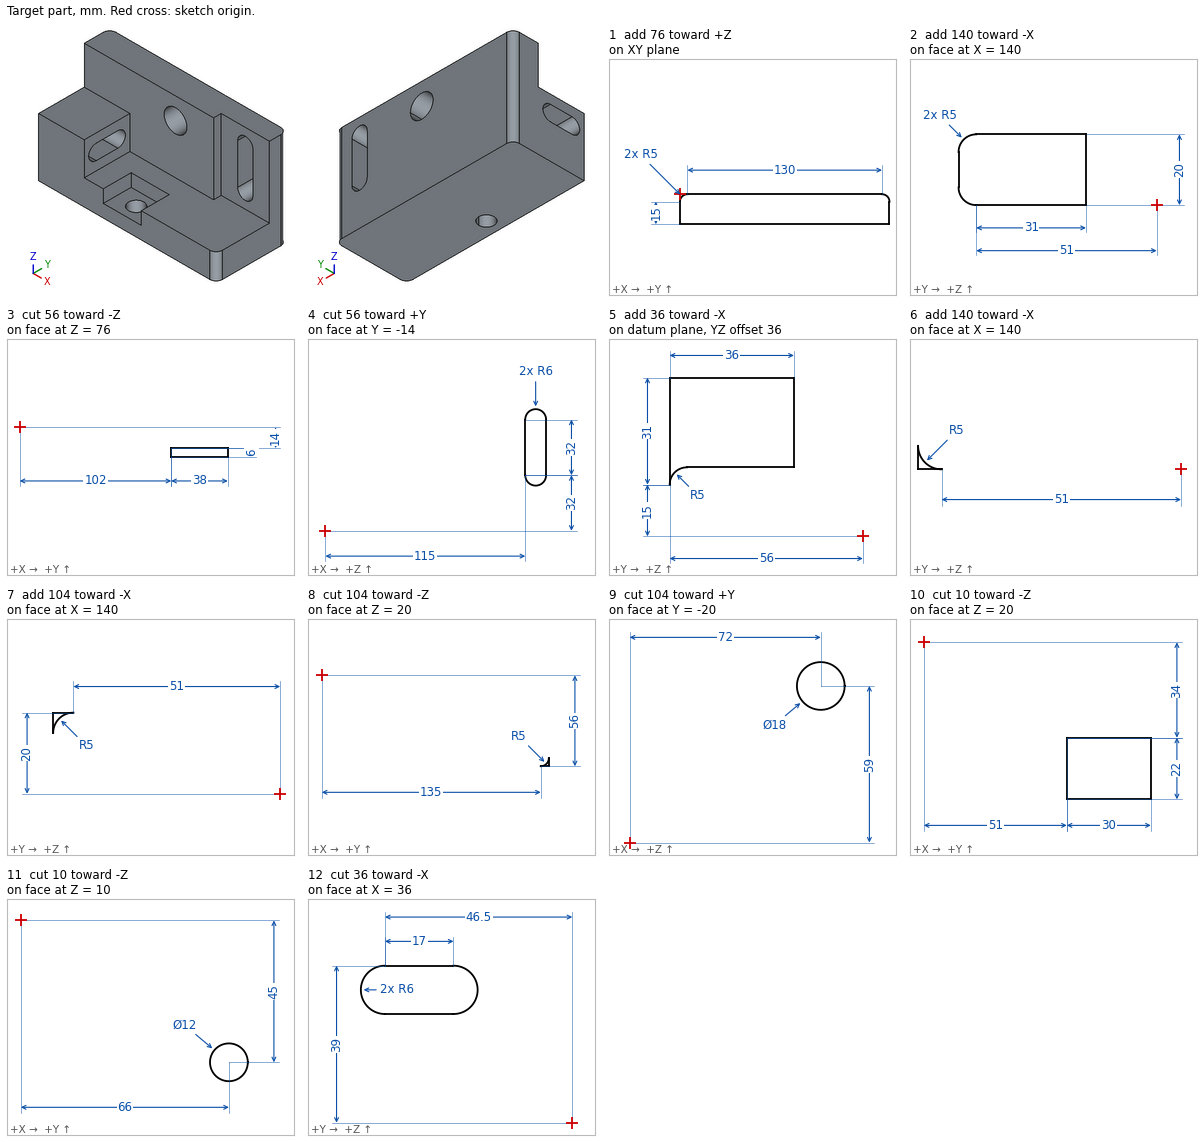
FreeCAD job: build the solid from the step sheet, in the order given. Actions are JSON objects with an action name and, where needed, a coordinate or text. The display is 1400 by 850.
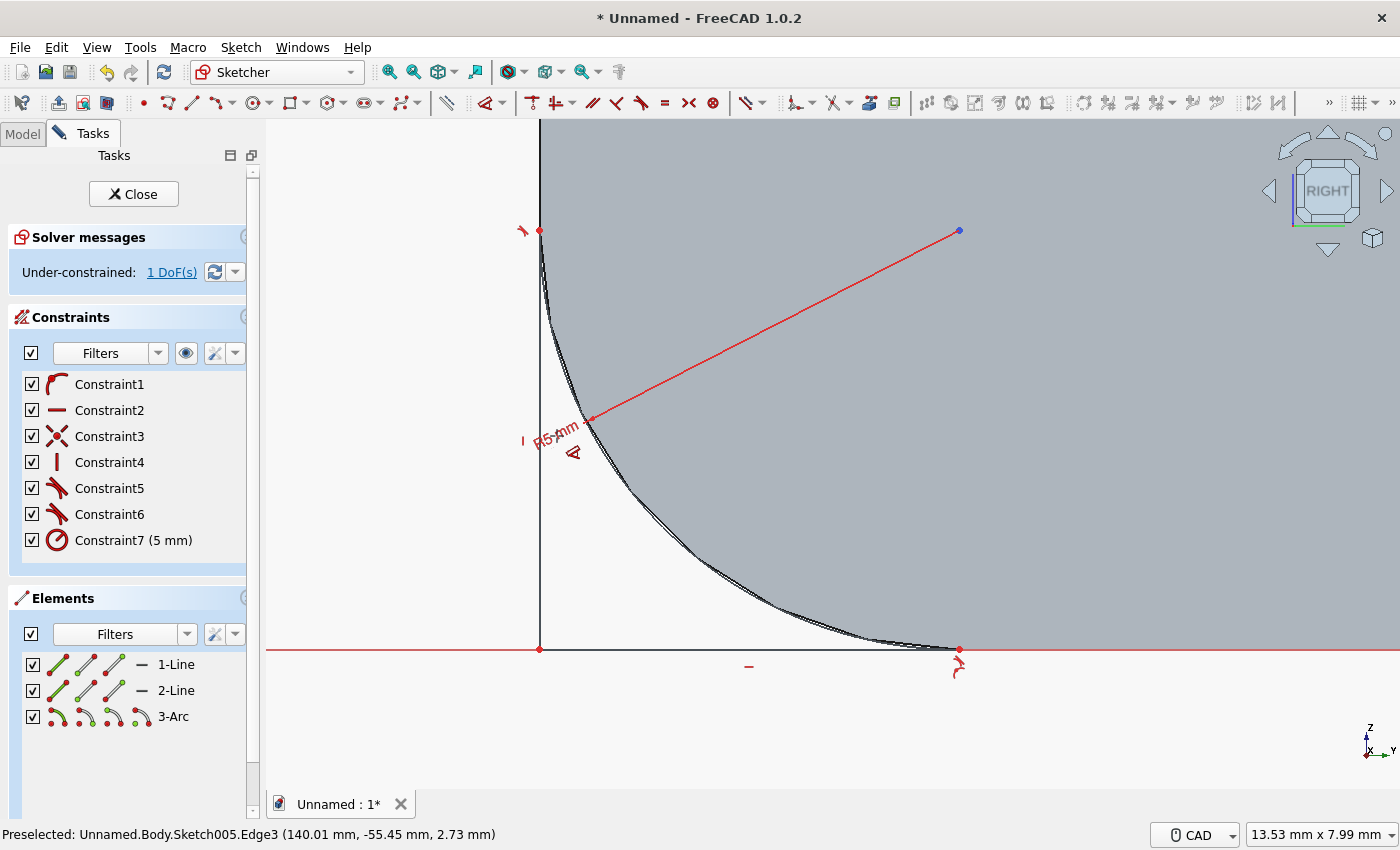
{"action": "left_click", "coordinate": [959, 650]}
{"action": "left_click", "coordinate": [1097, 684]}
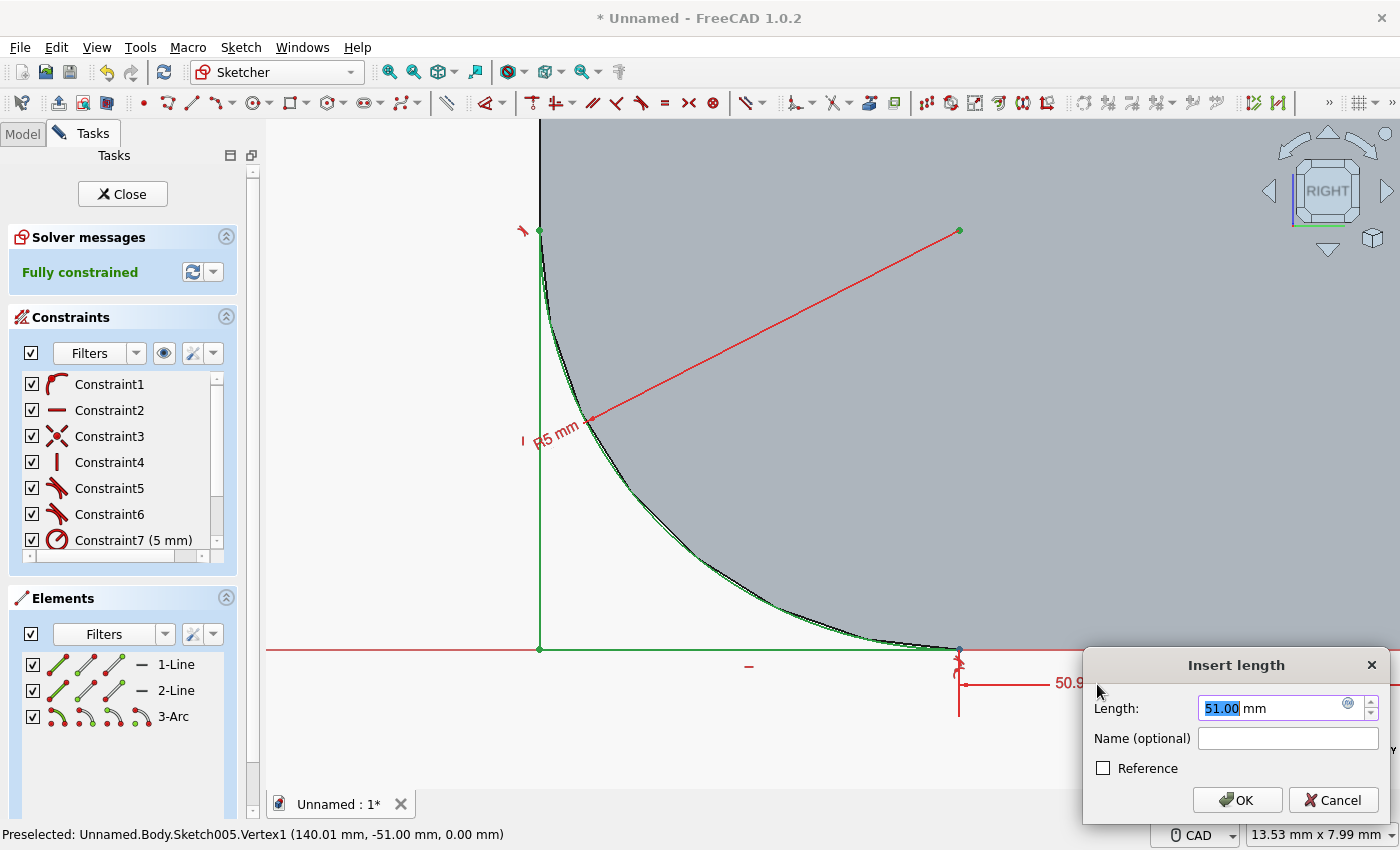
{"action": "type", "text": "51"}
{"action": "key", "text": "Return"}
{"action": "key", "text": "Escape"}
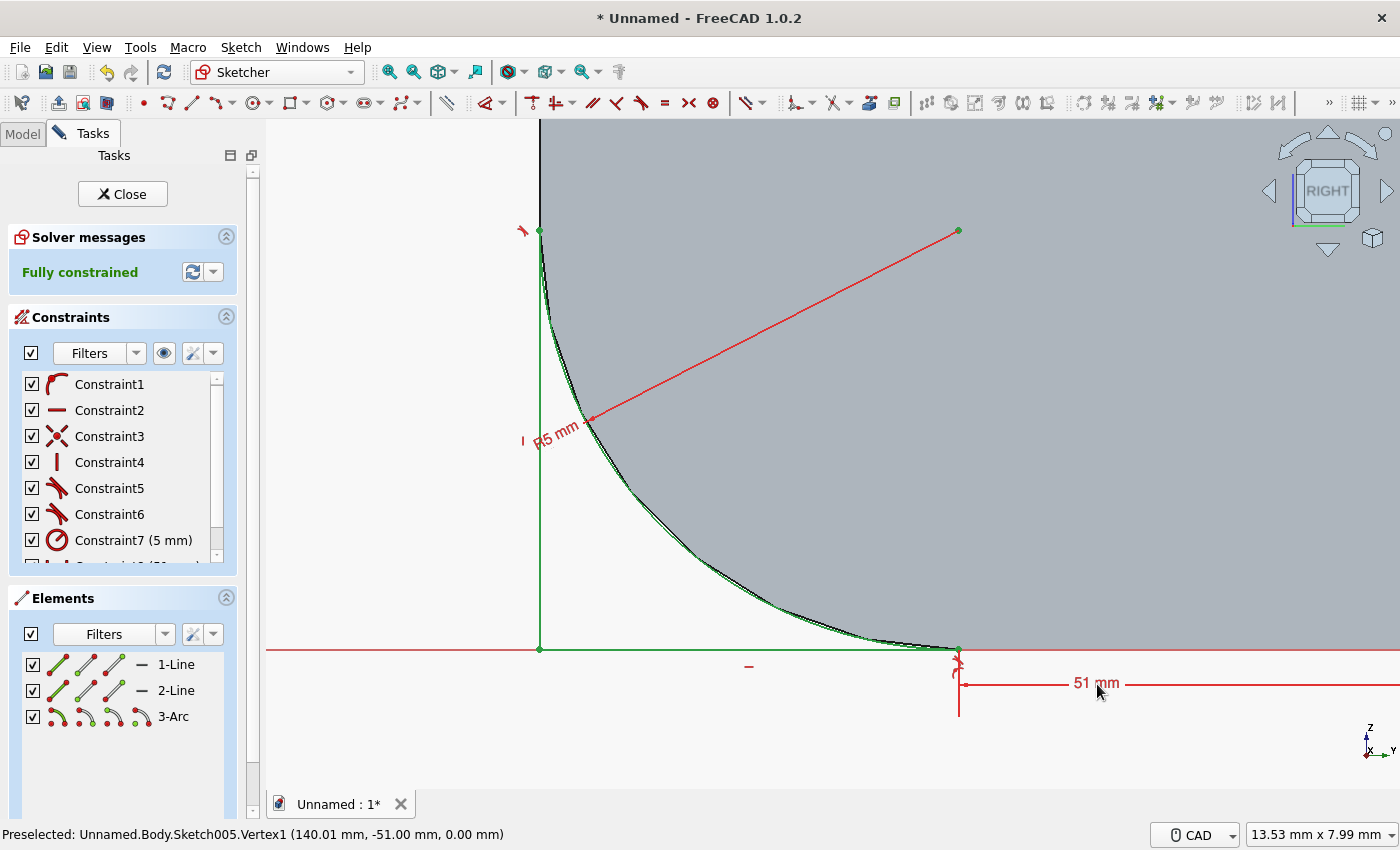
{"action": "left_click", "coordinate": [123, 194]}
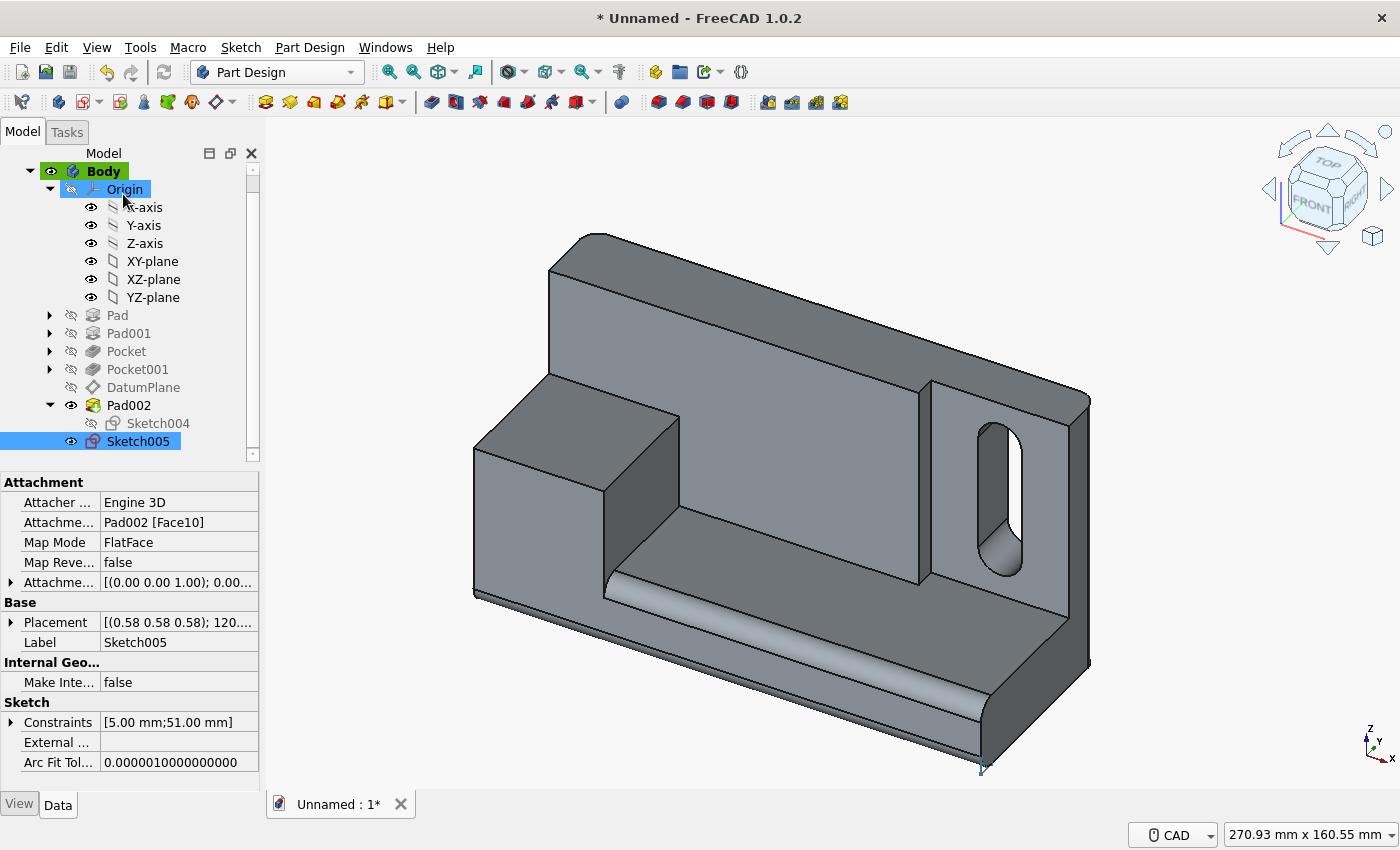
{"action": "left_click", "coordinate": [266, 102]}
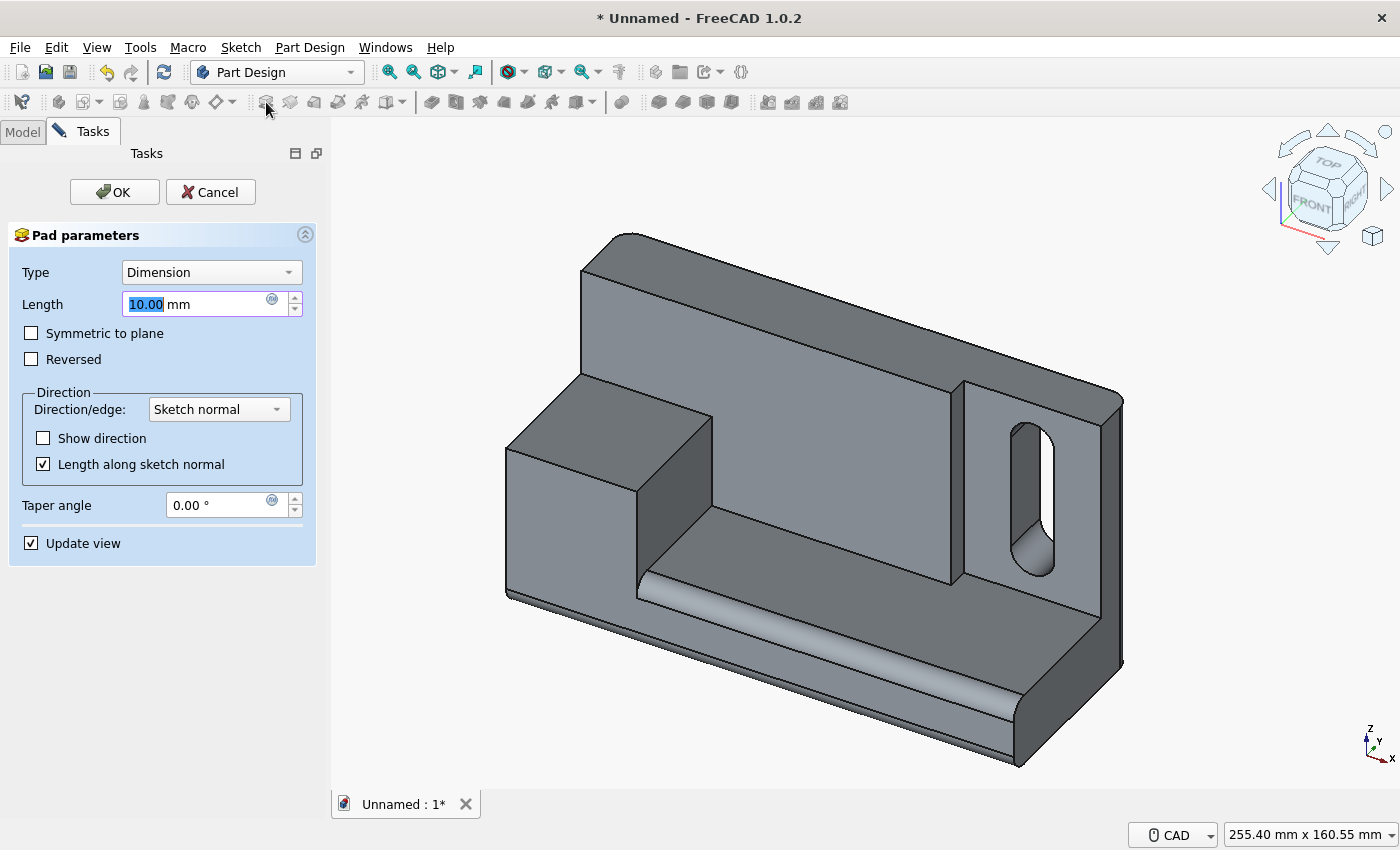
{"action": "type", "text": "140"}
{"action": "key", "text": "Tab"}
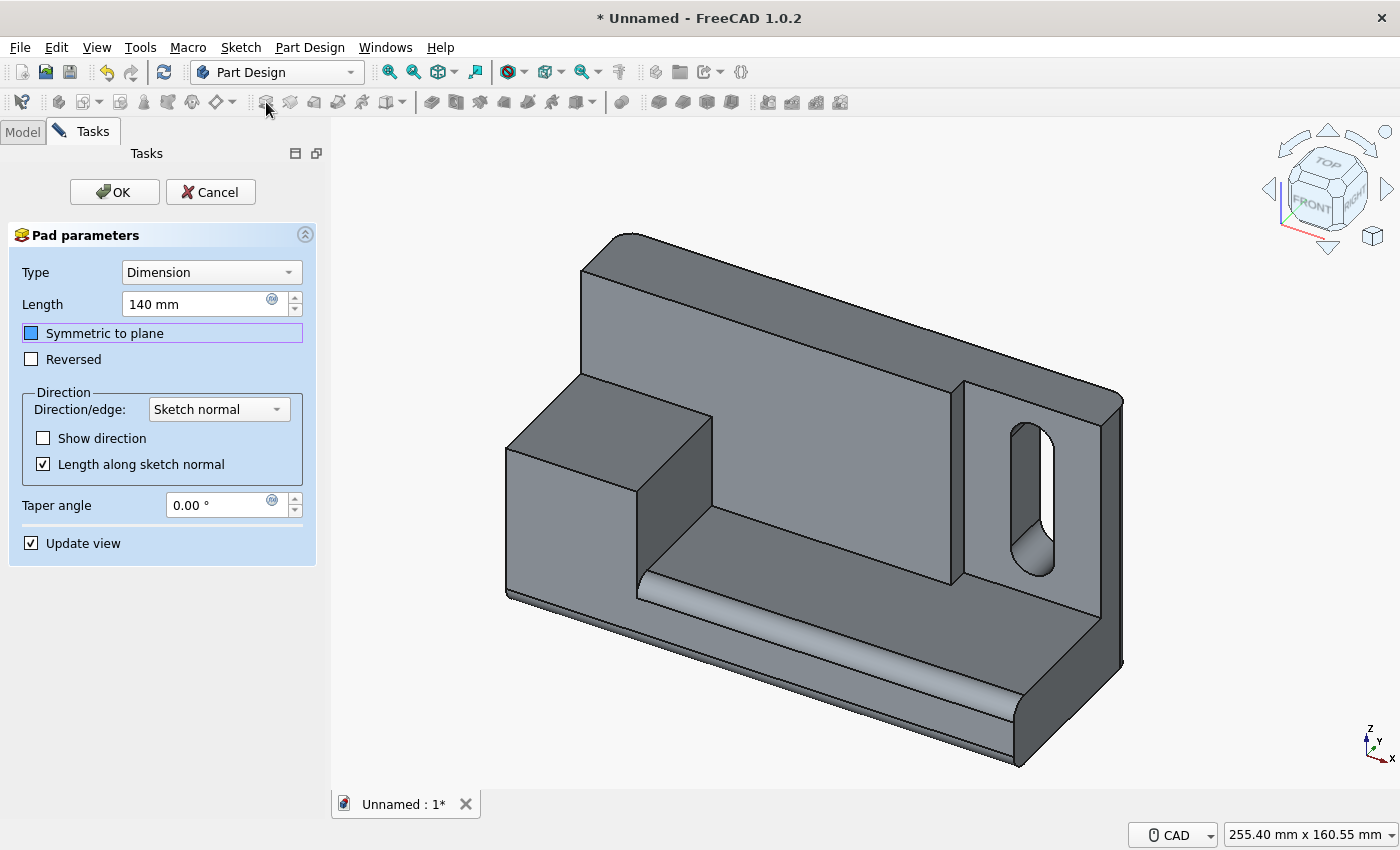
{"action": "left_click", "coordinate": [30, 359]}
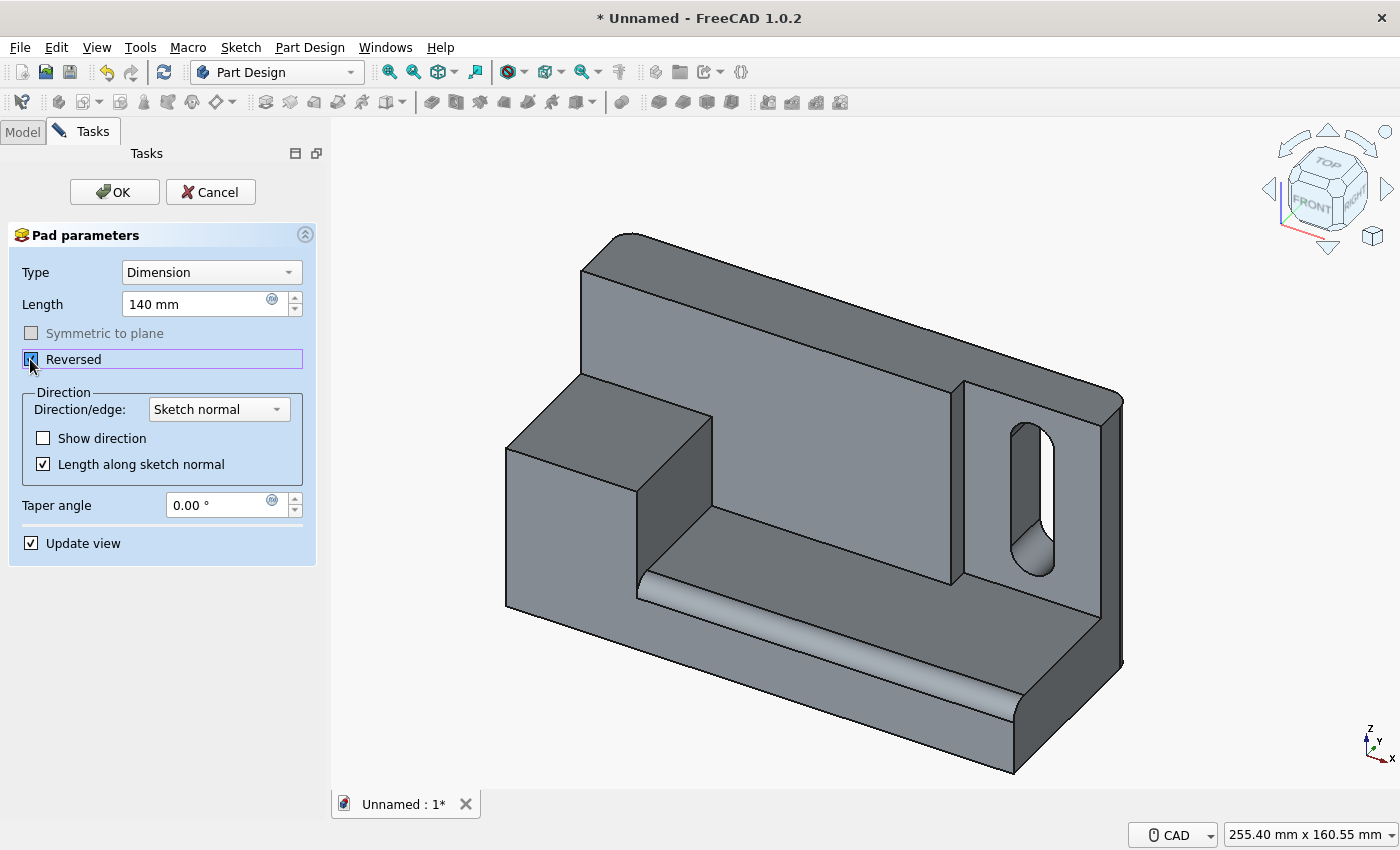
{"action": "left_click", "coordinate": [115, 192]}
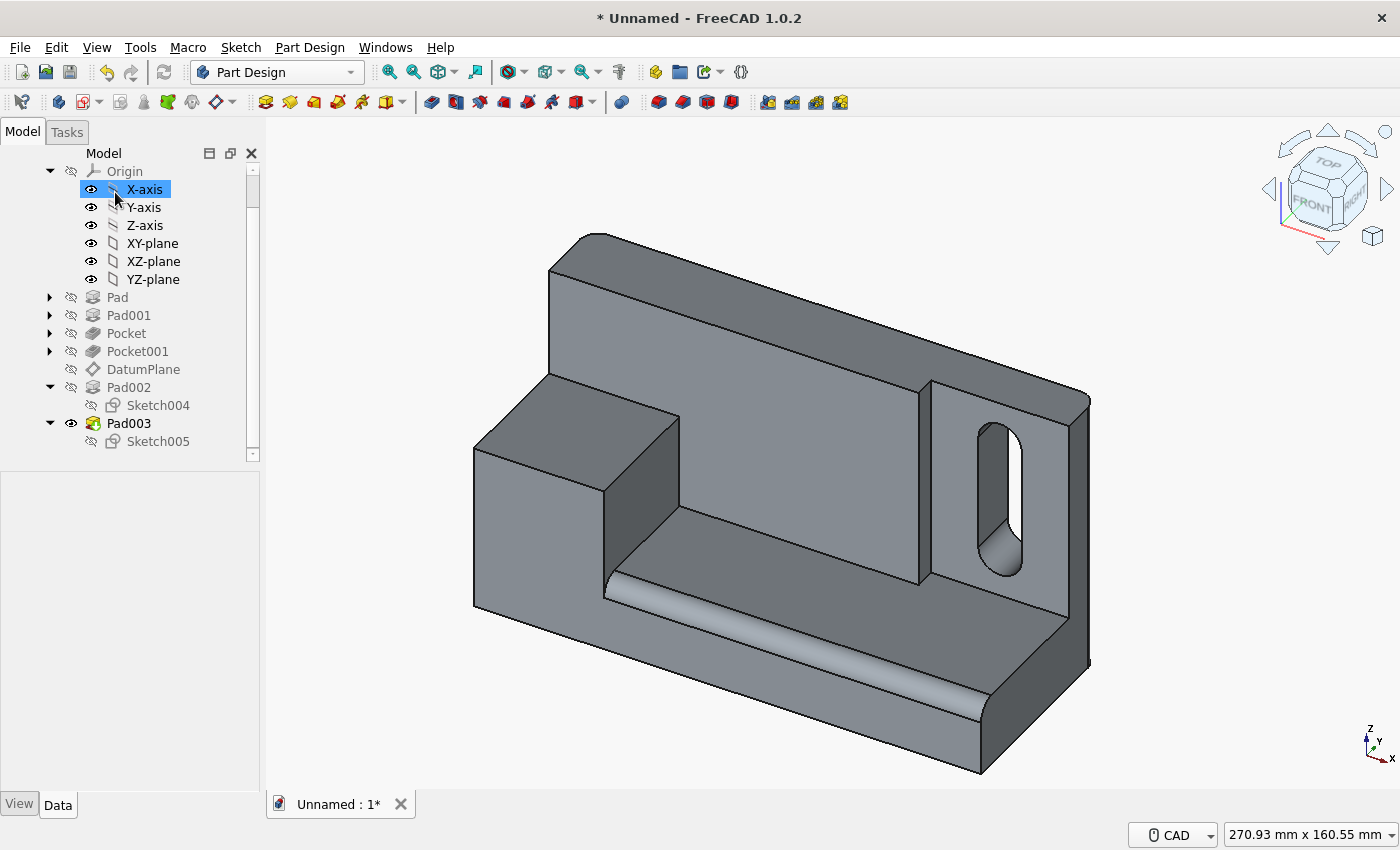
{"action": "left_click", "coordinate": [1065, 671]}